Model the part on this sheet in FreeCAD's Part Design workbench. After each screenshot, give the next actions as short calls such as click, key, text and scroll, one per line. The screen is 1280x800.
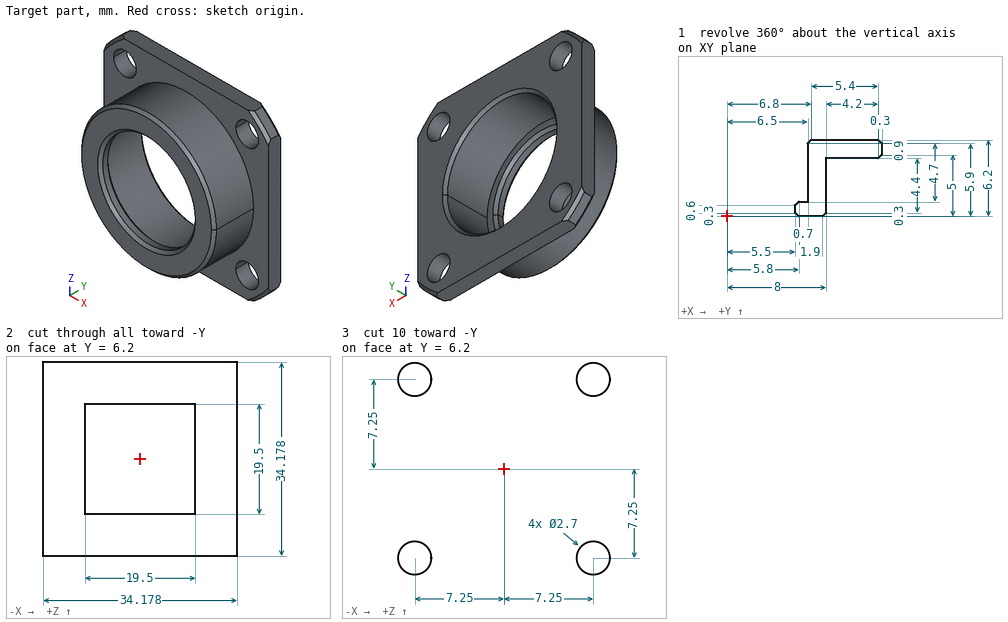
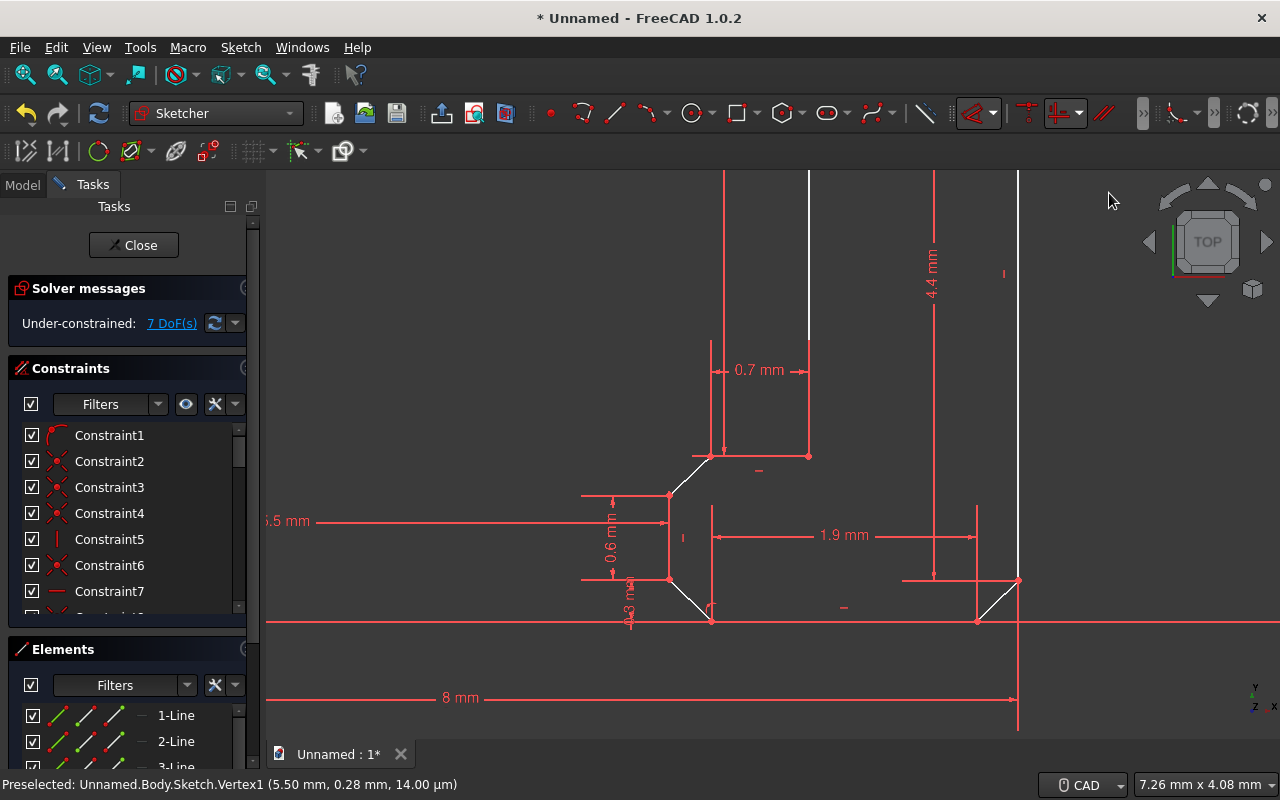
click(712, 622)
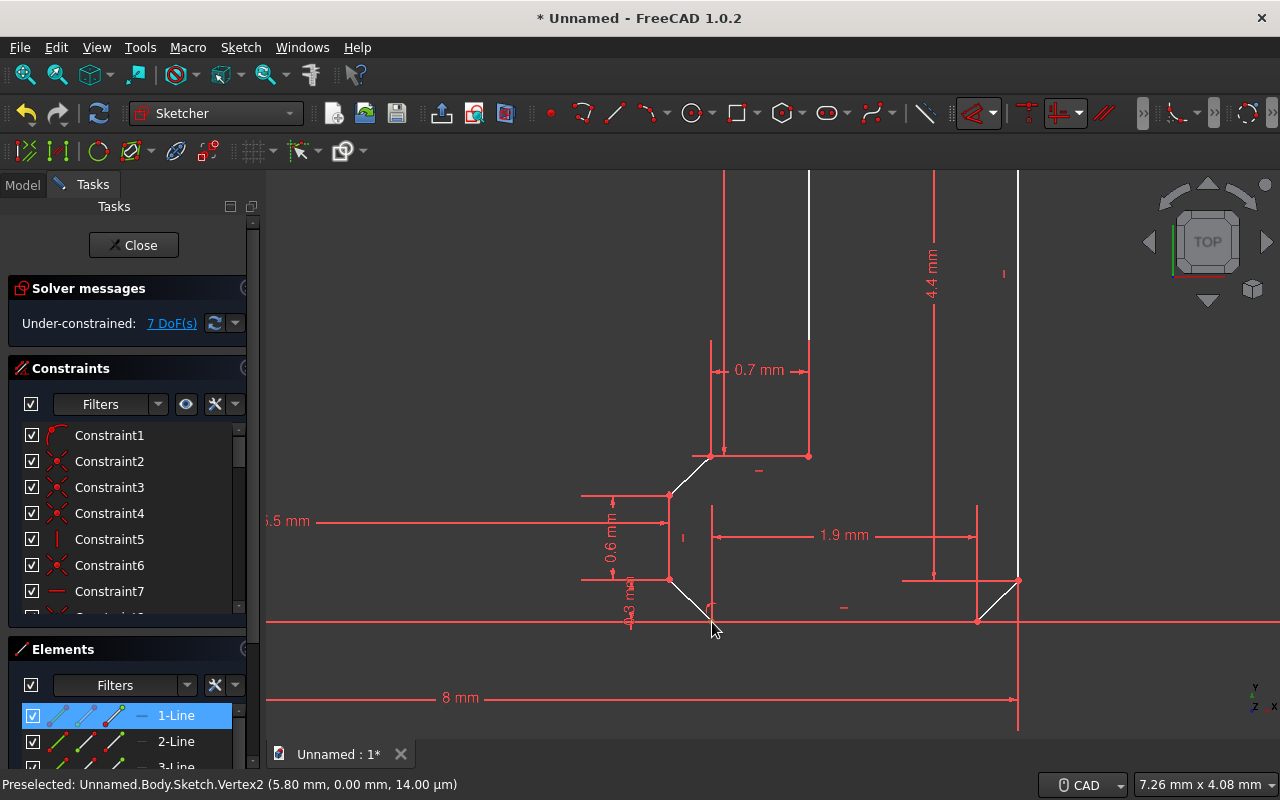
click(996, 114)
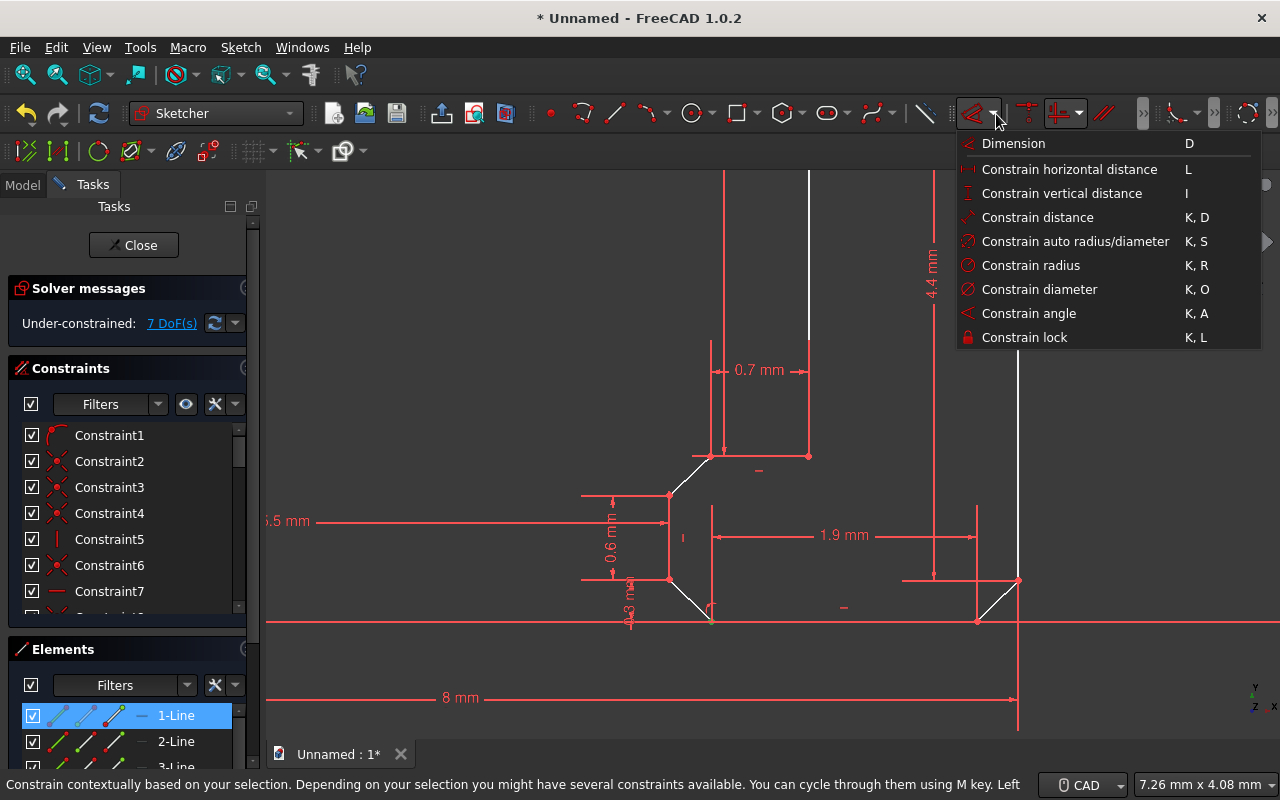
click(1109, 169)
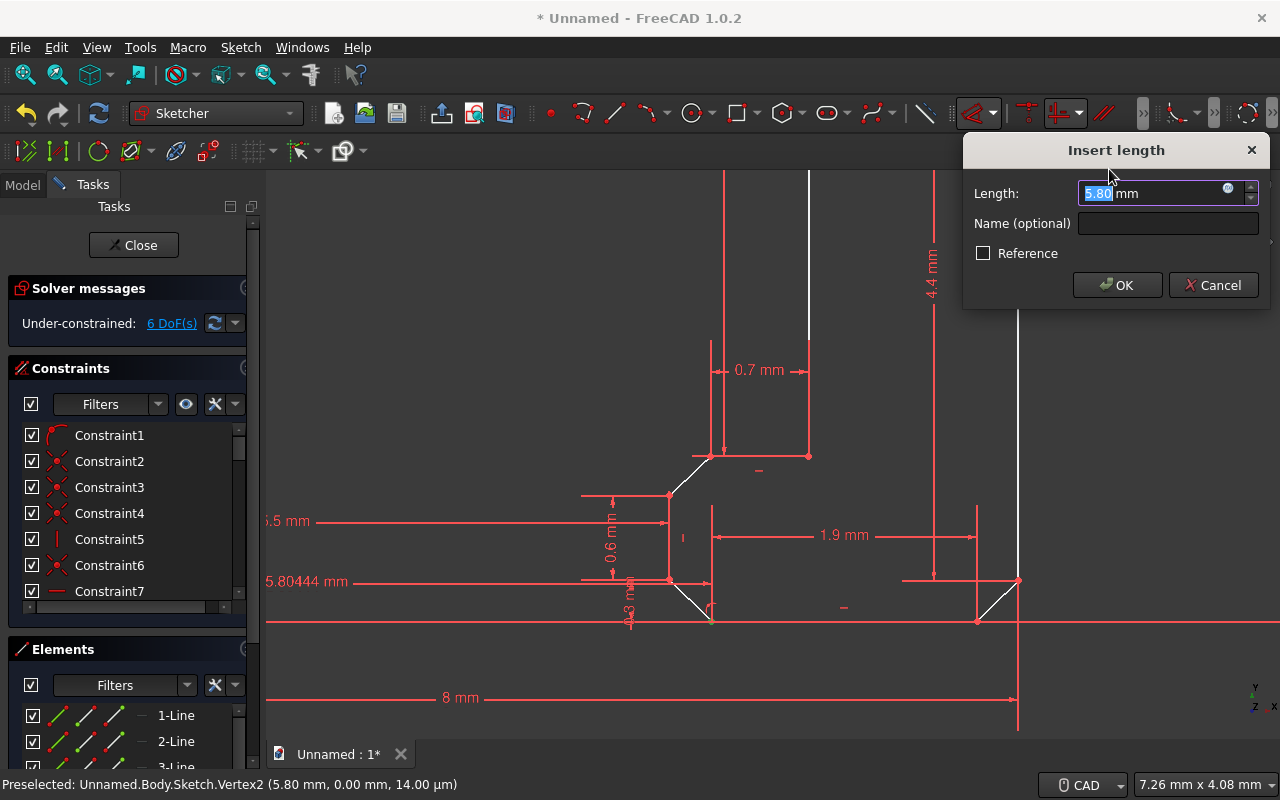
text(5.8)
key(Return)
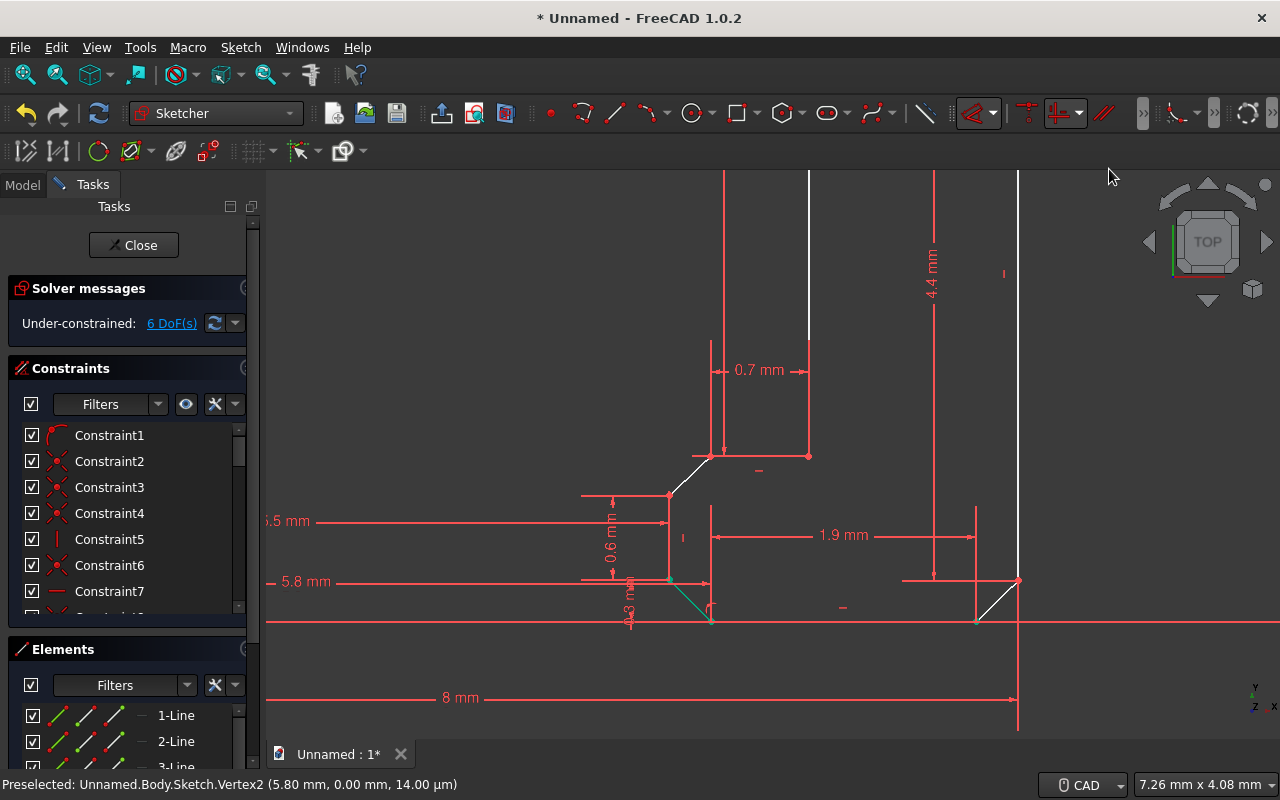
click(1018, 581)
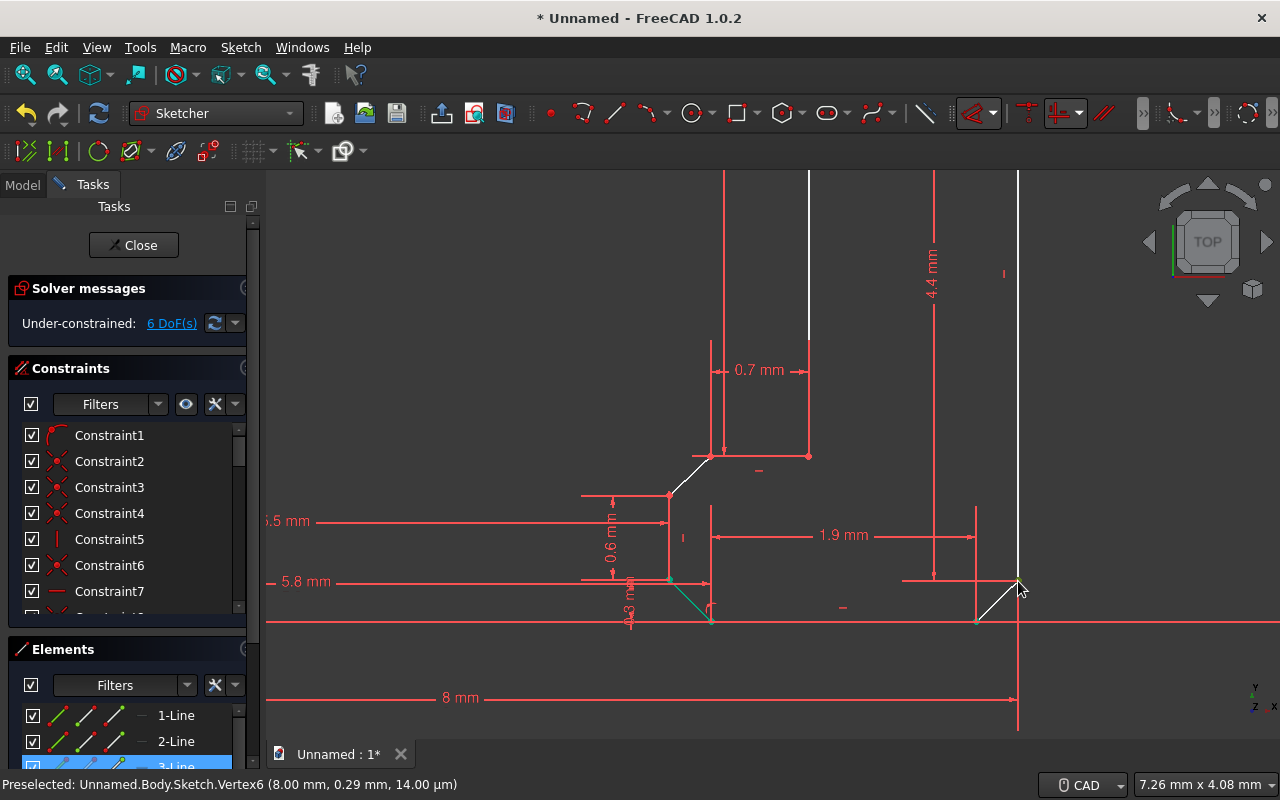
click(996, 114)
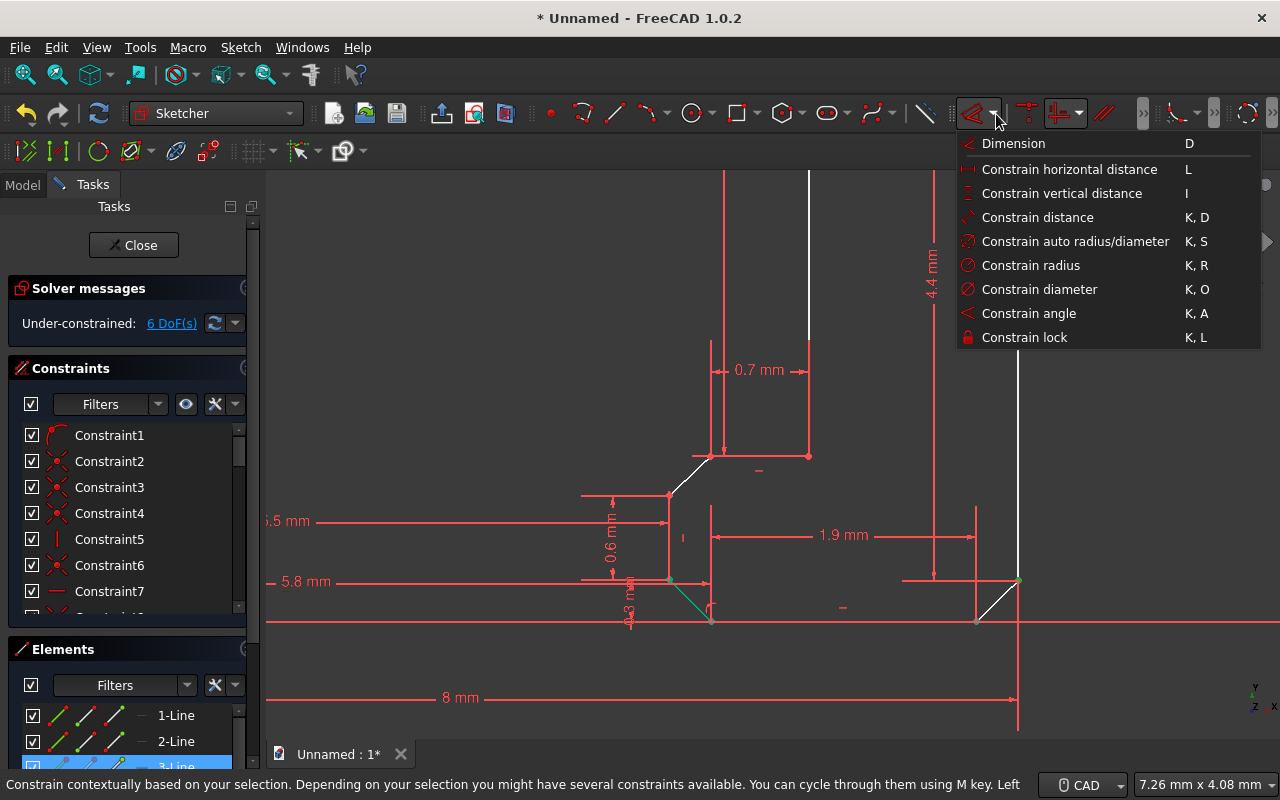
click(1109, 193)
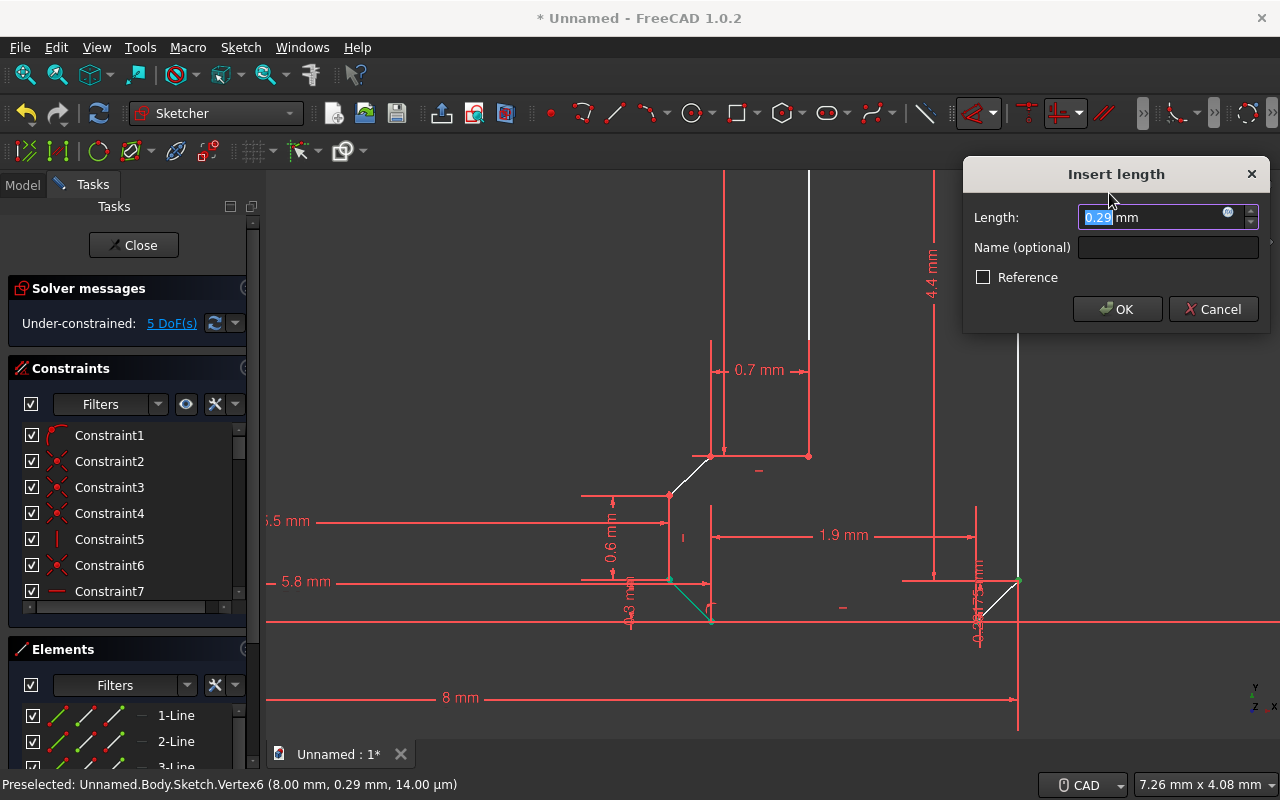
text(0.3)
key(Return)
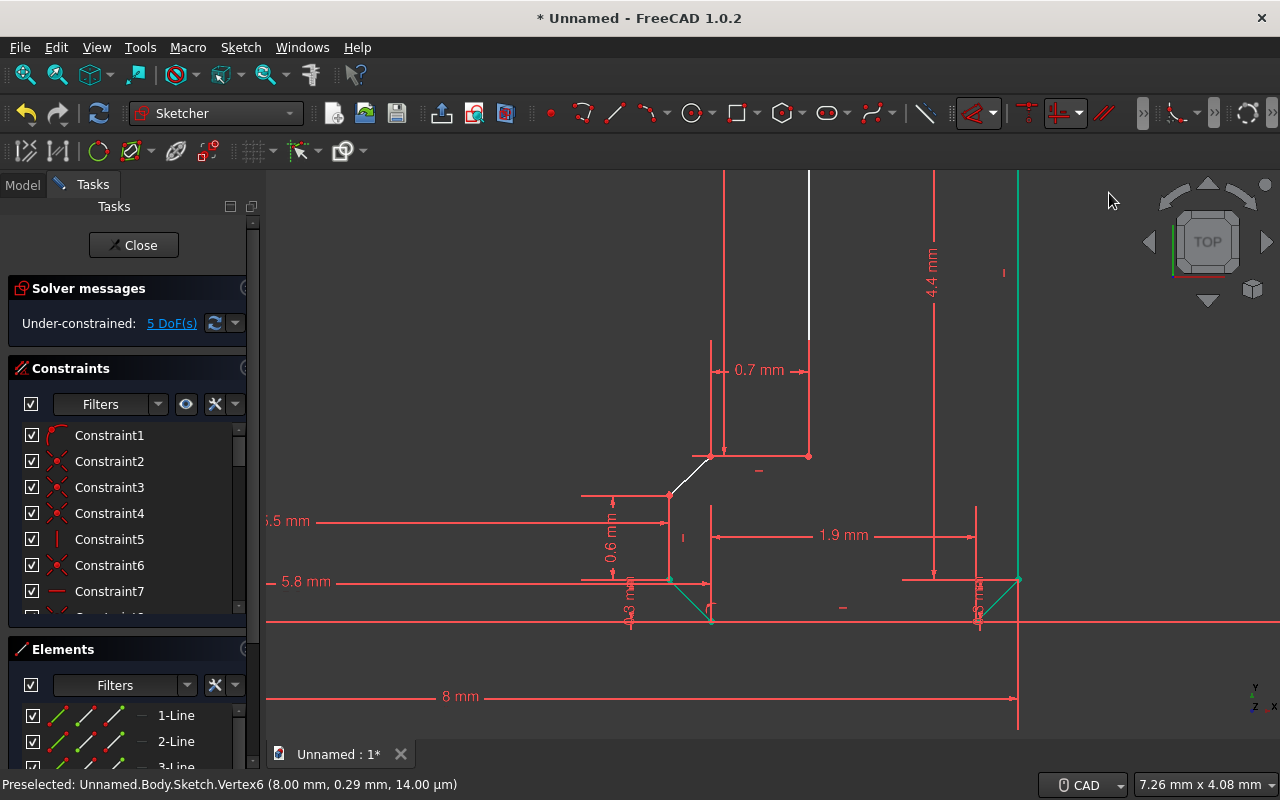
scroll(675, 569, down, 6)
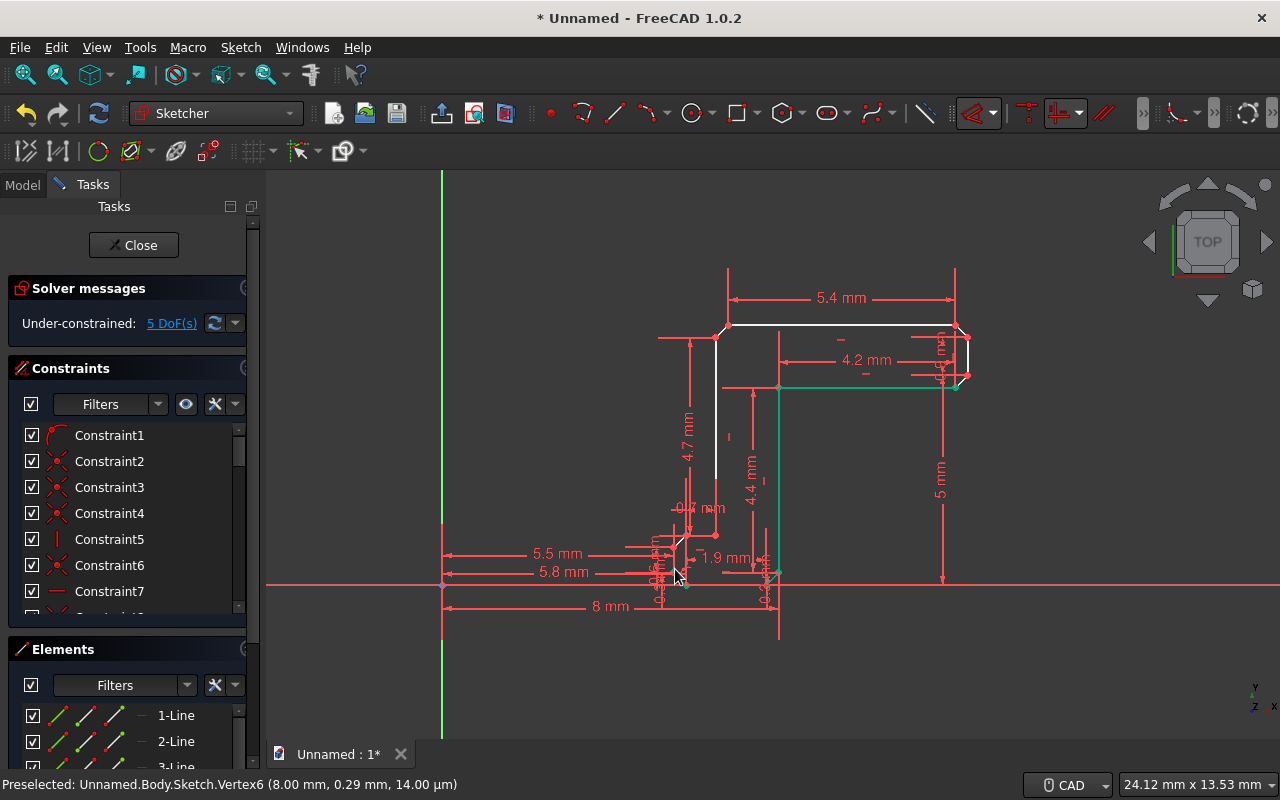
click(955, 325)